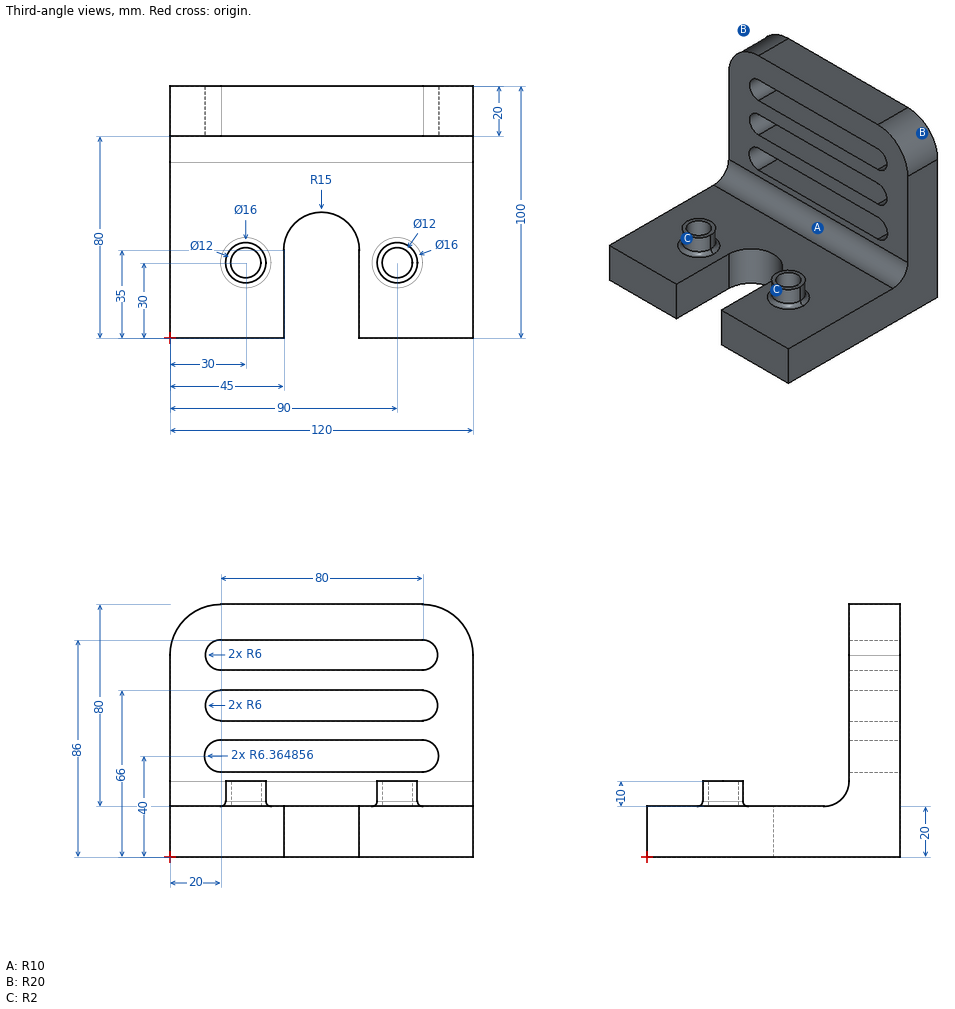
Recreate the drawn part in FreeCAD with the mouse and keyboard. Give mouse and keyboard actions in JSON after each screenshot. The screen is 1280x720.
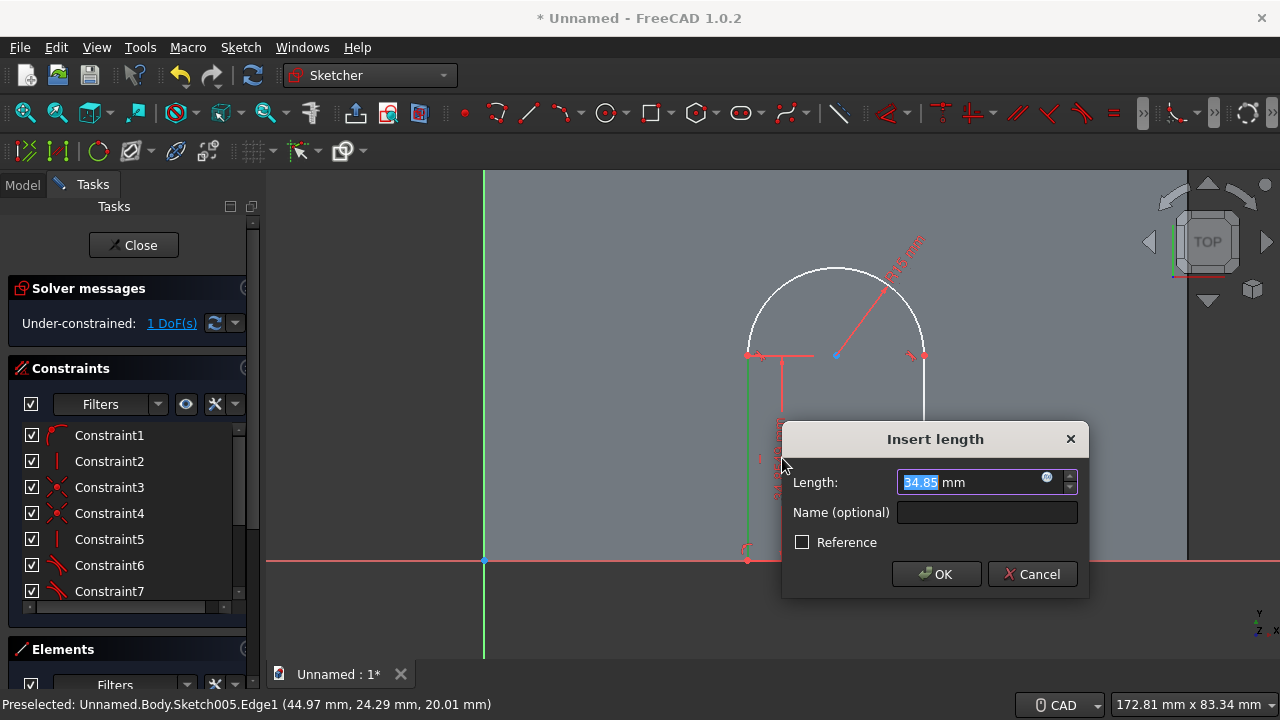
{"action": "type", "text": "35"}
{"action": "key", "text": "Return"}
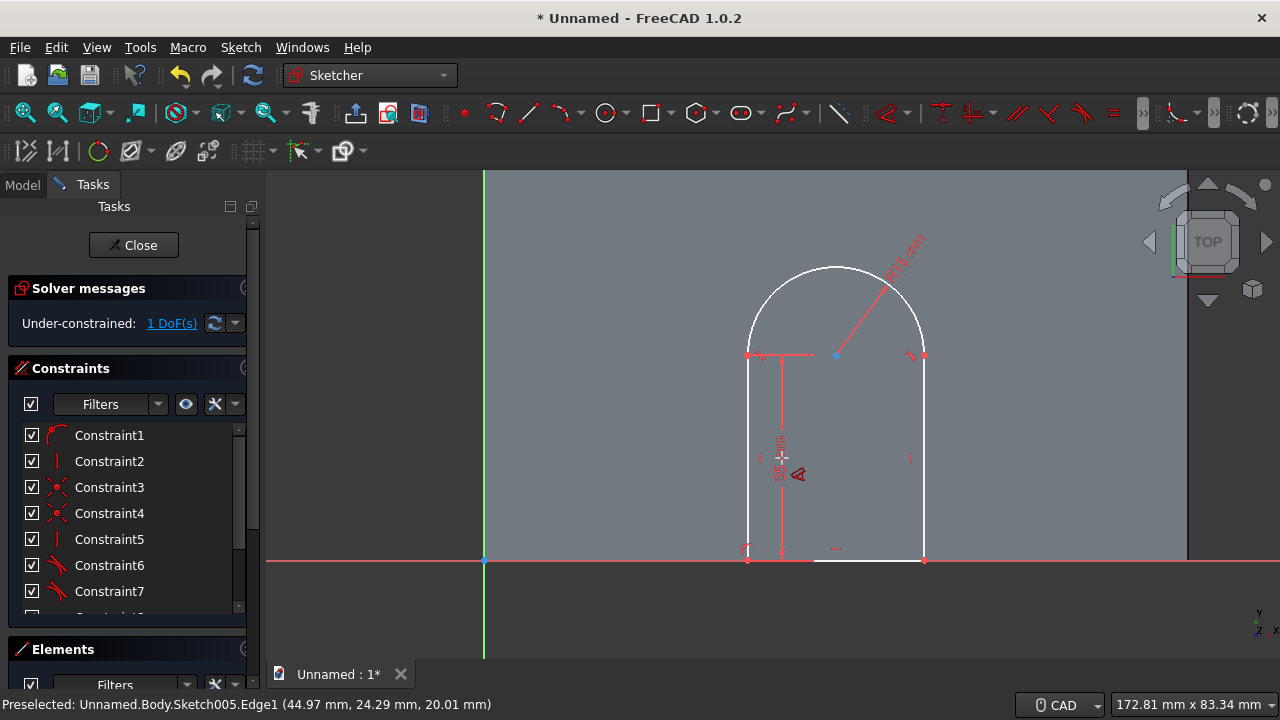
{"action": "left_click", "coordinate": [748, 355]}
{"action": "left_click", "coordinate": [616, 595]}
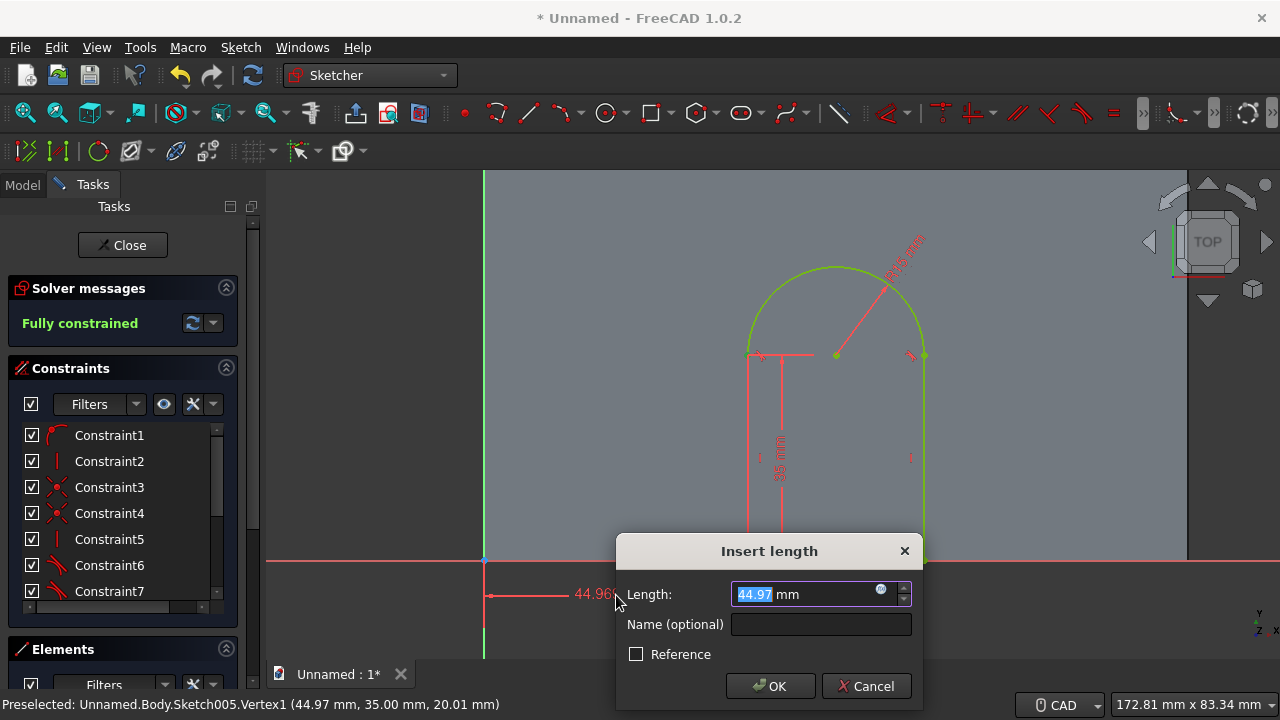
{"action": "type", "text": "45"}
{"action": "key", "text": "Return"}
{"action": "key", "text": "Escape"}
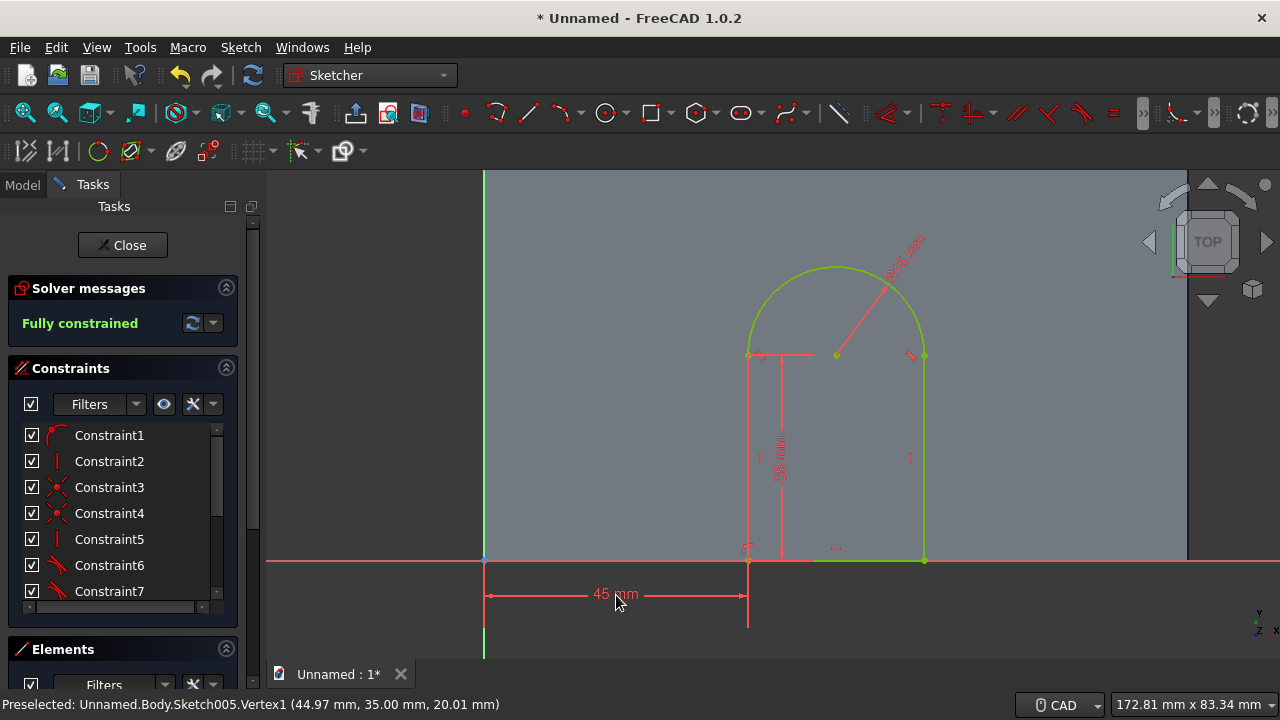
{"action": "left_click", "coordinate": [123, 245]}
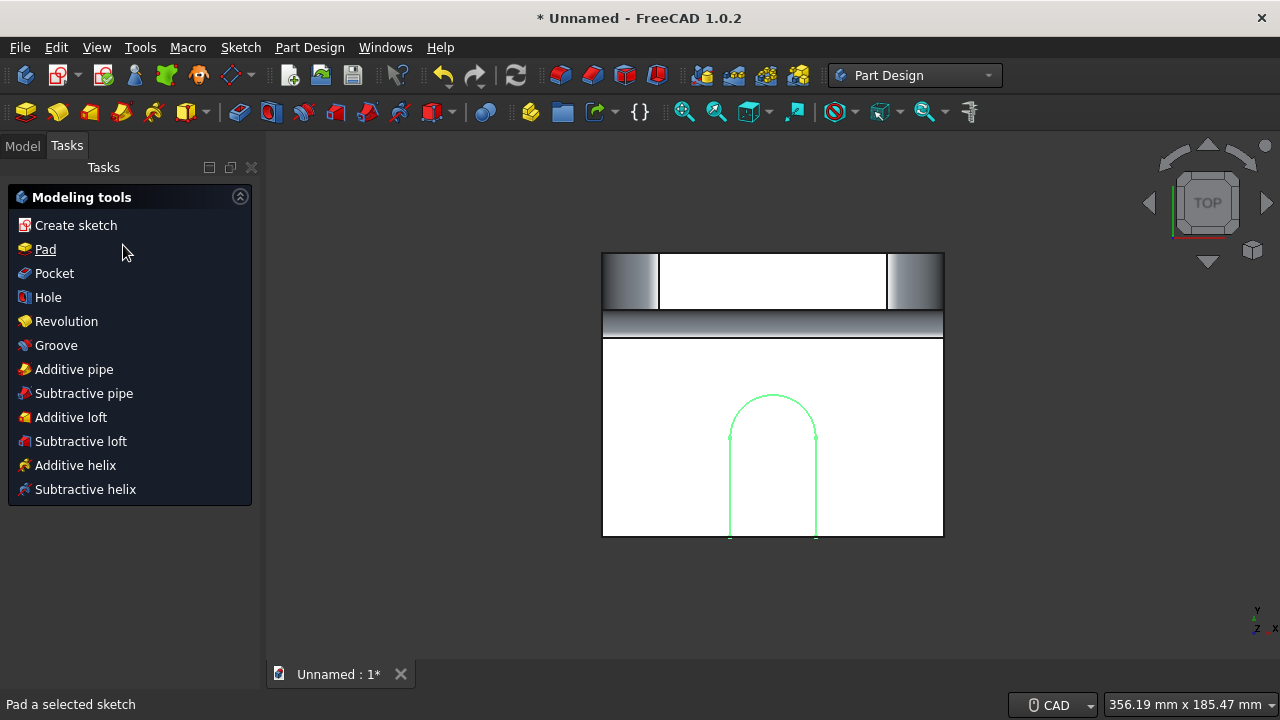
{"action": "left_click", "coordinate": [240, 112]}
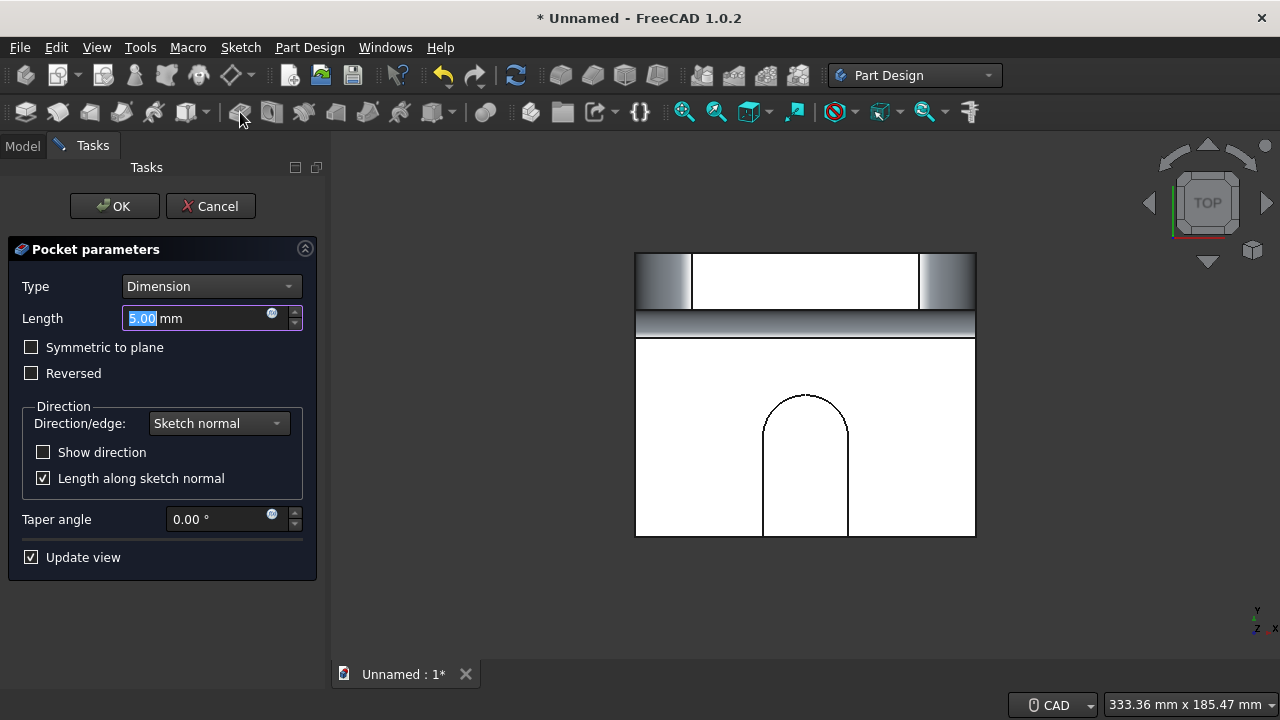
{"action": "left_click", "coordinate": [212, 286]}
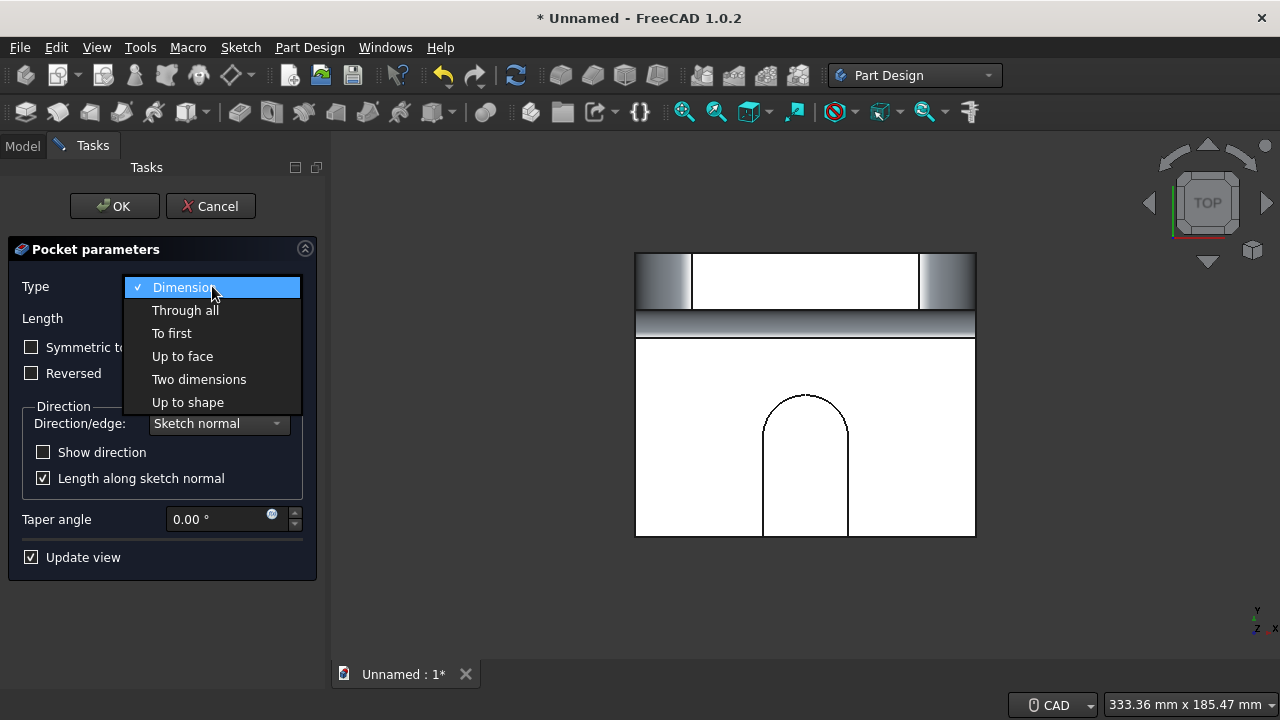
{"action": "left_click", "coordinate": [212, 310]}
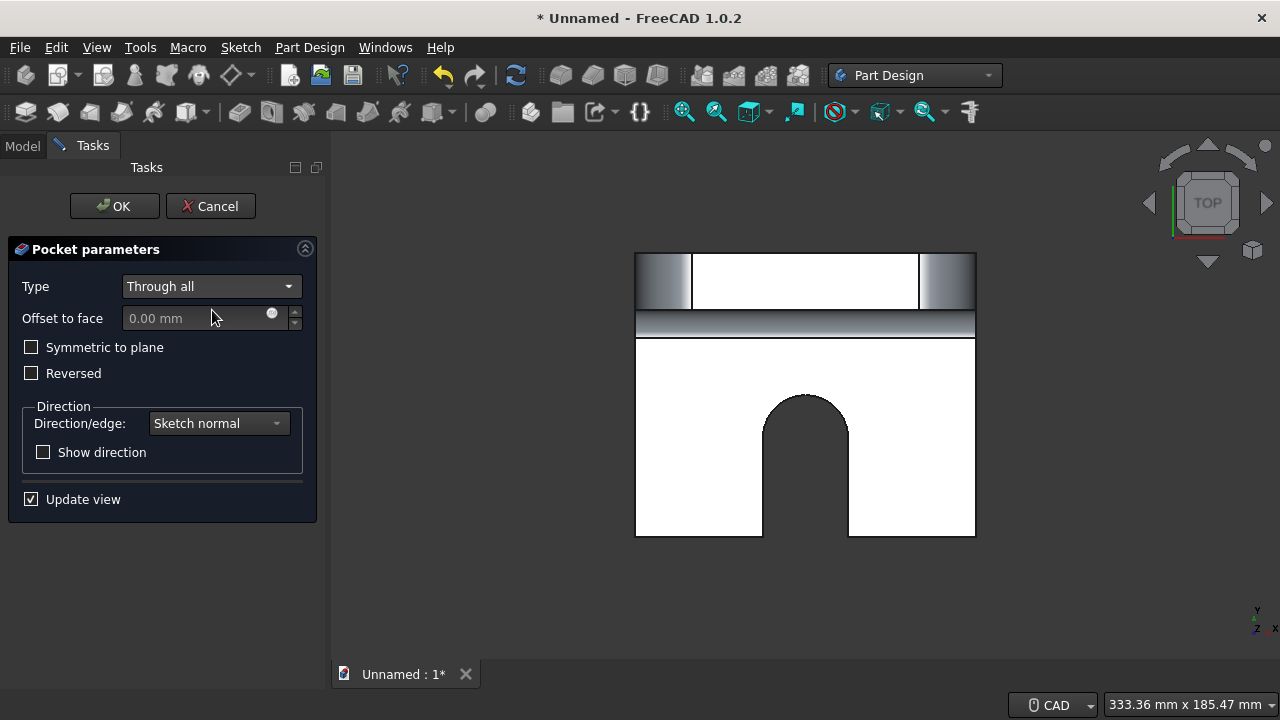
{"action": "left_click", "coordinate": [115, 206]}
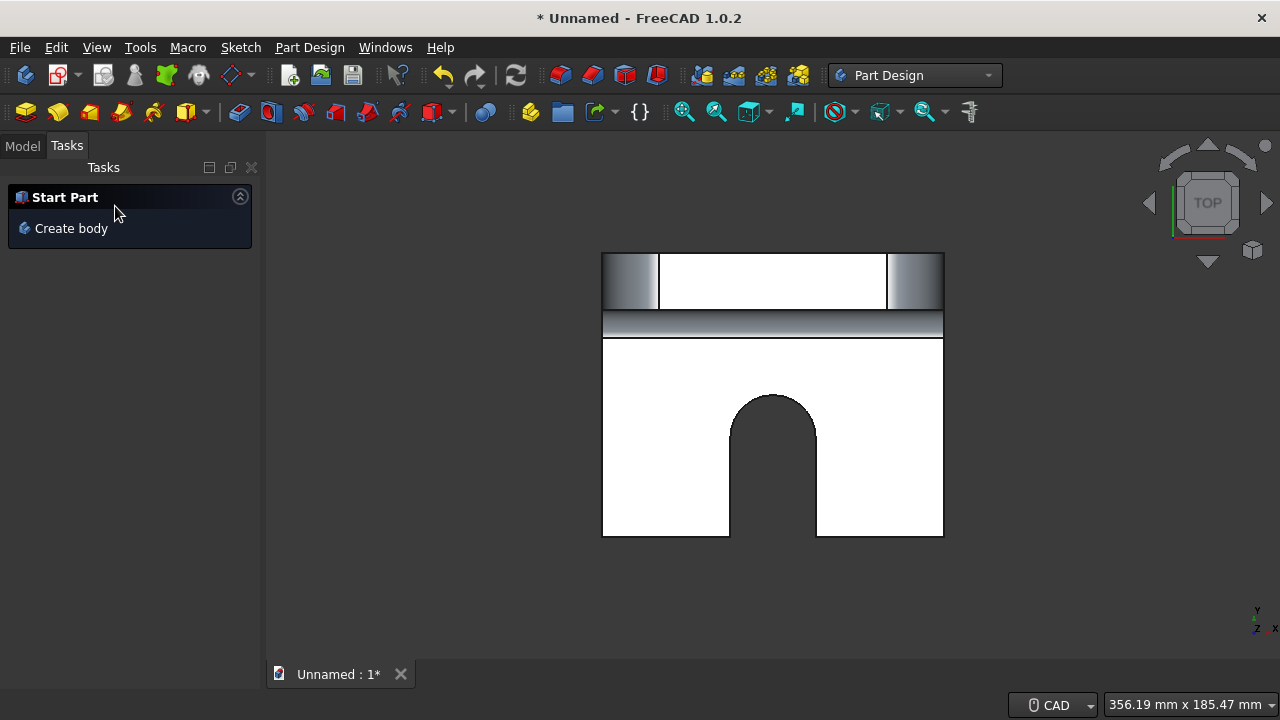
{"action": "left_click", "coordinate": [871, 408]}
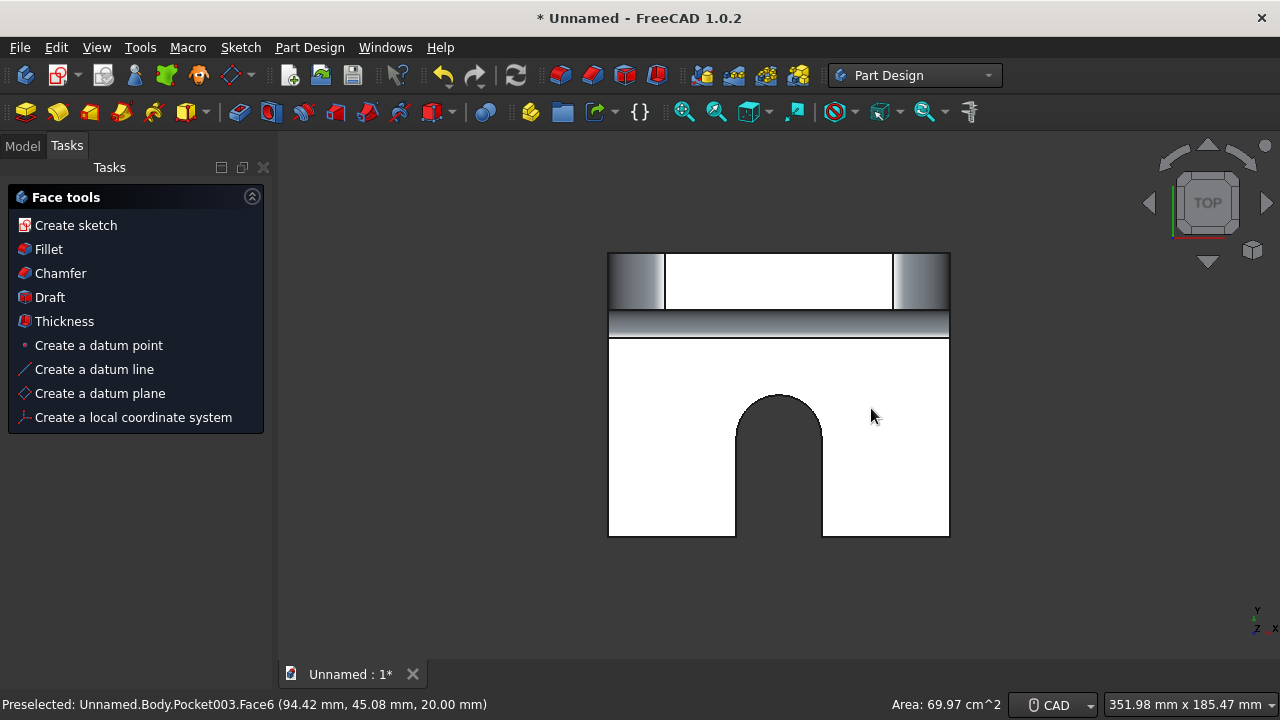
{"action": "left_click", "coordinate": [58, 76]}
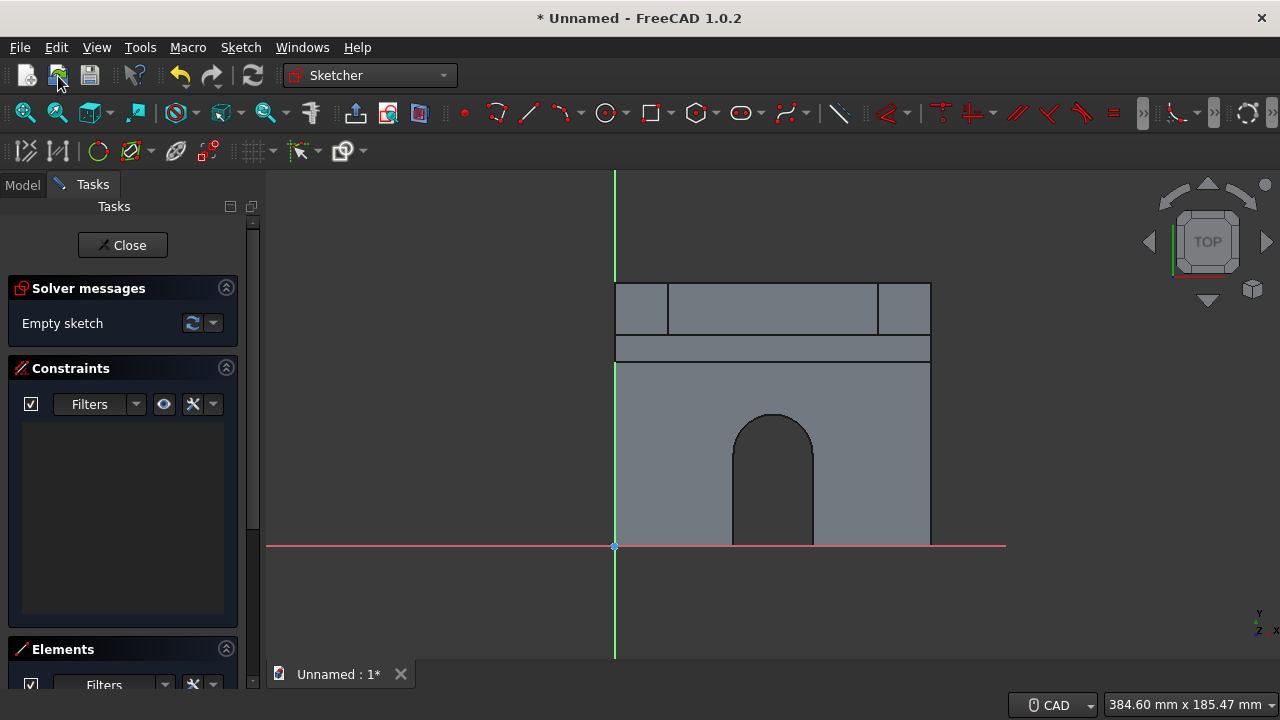
{"action": "left_click", "coordinate": [420, 114]}